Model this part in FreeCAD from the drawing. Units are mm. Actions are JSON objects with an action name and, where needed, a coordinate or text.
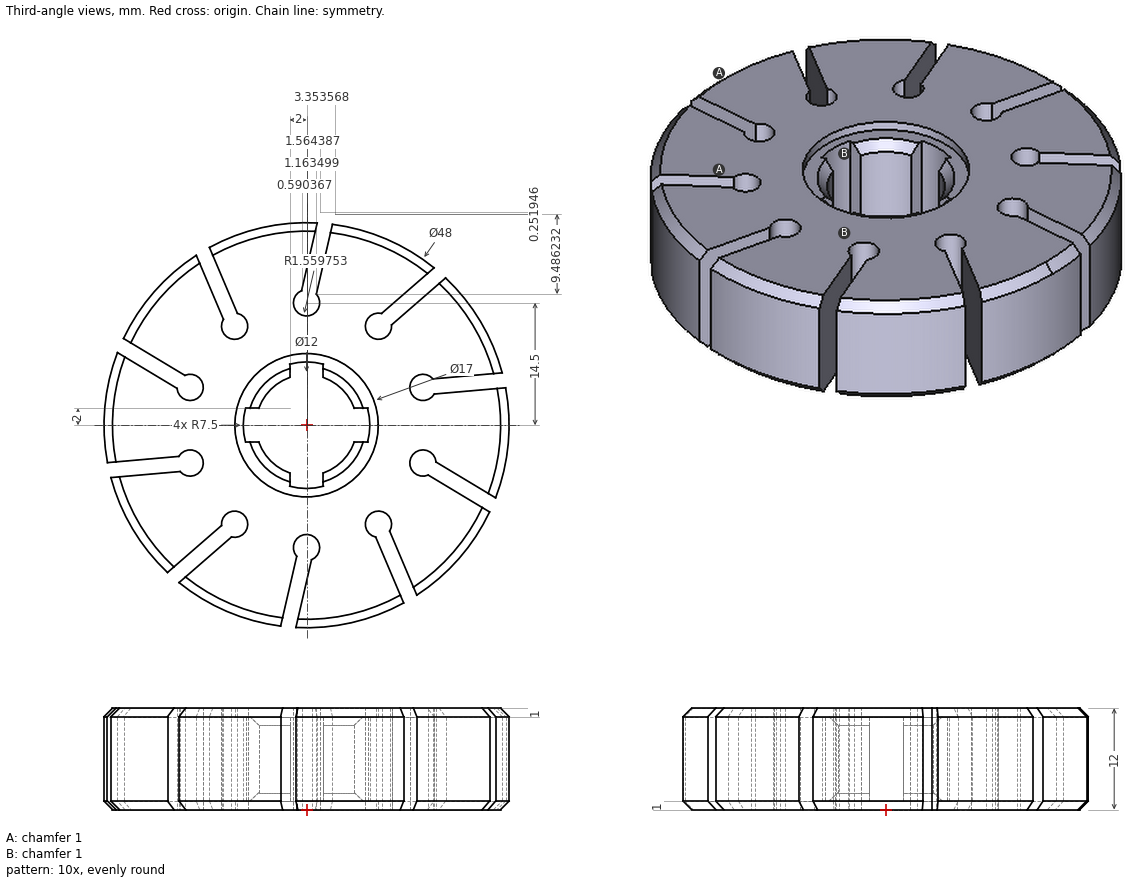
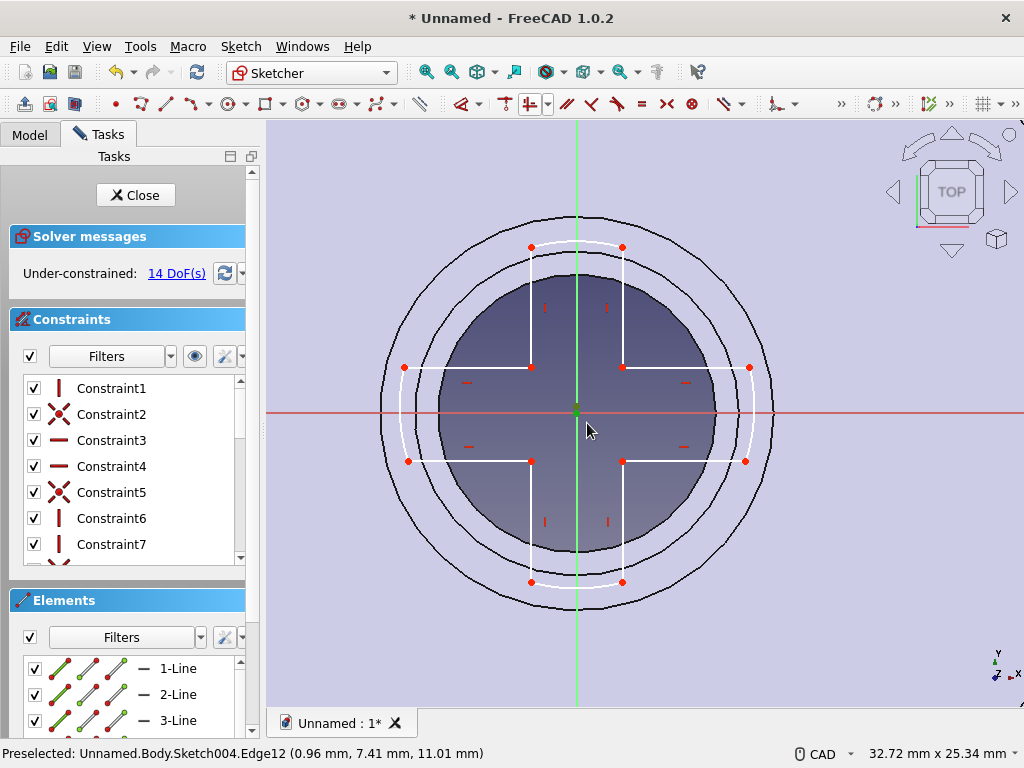
{"action": "left_click", "coordinate": [505, 104]}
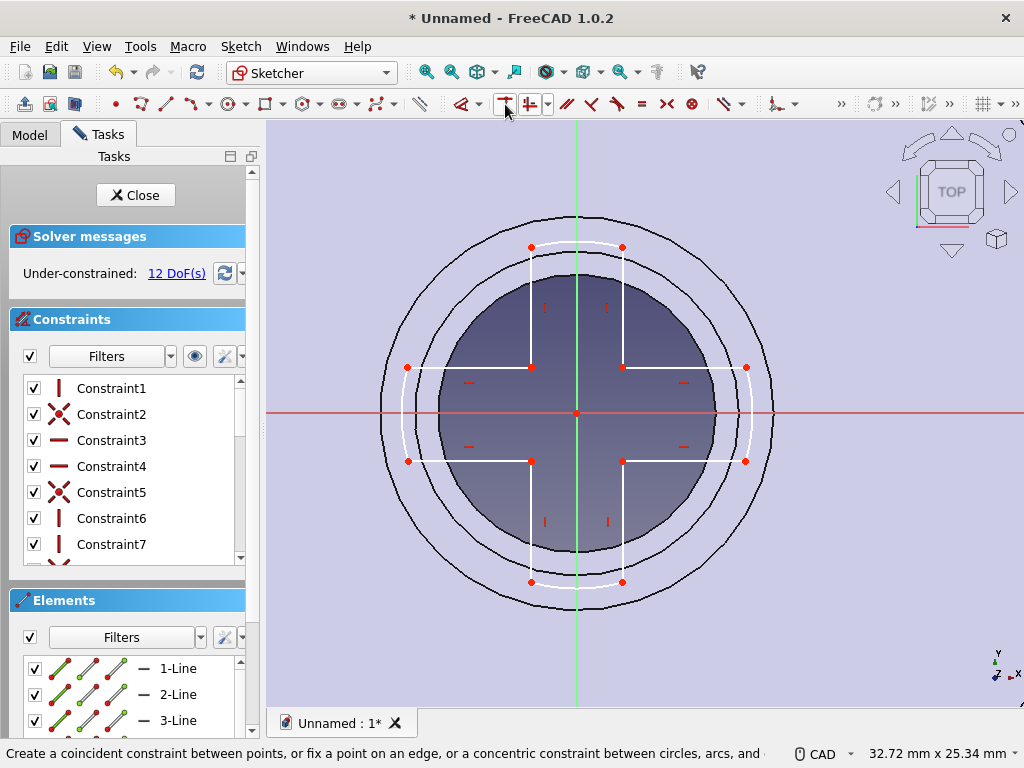
{"action": "left_click", "coordinate": [403, 396]}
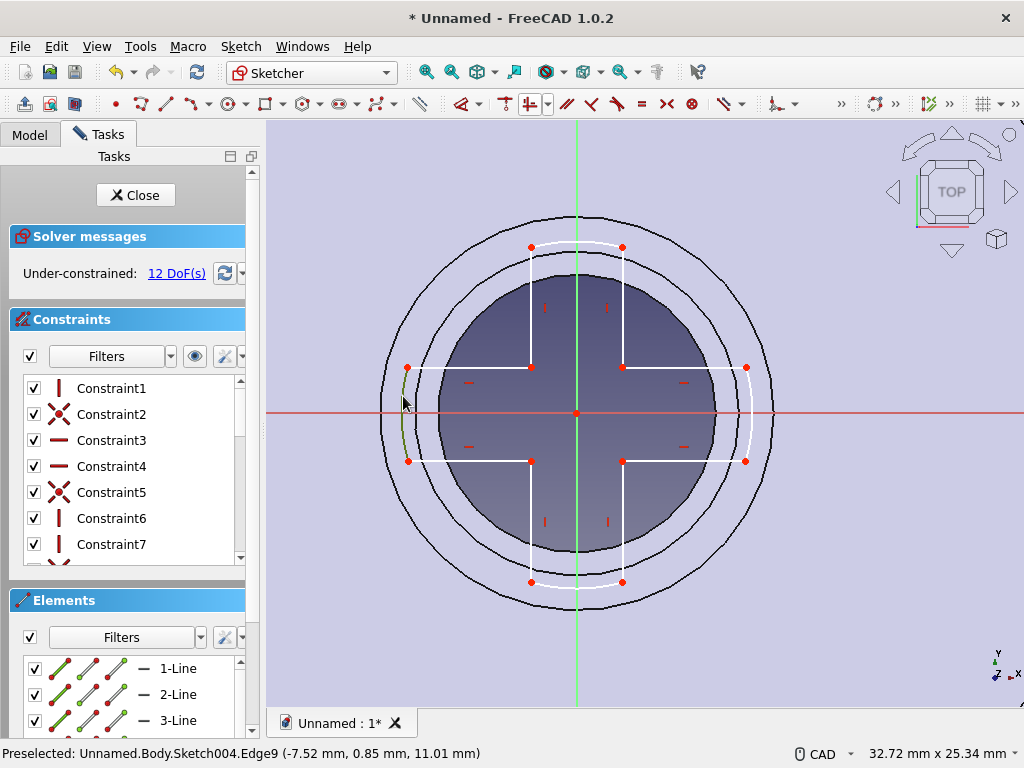
{"action": "left_click", "coordinate": [558, 588]}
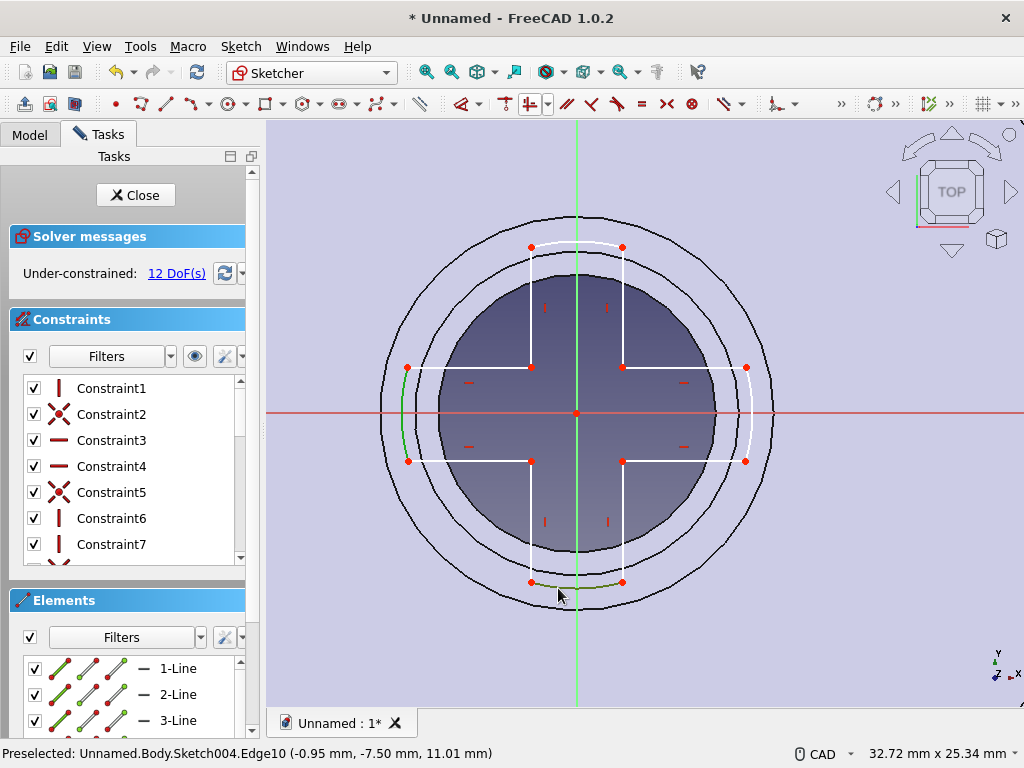
{"action": "left_click", "coordinate": [751, 433]}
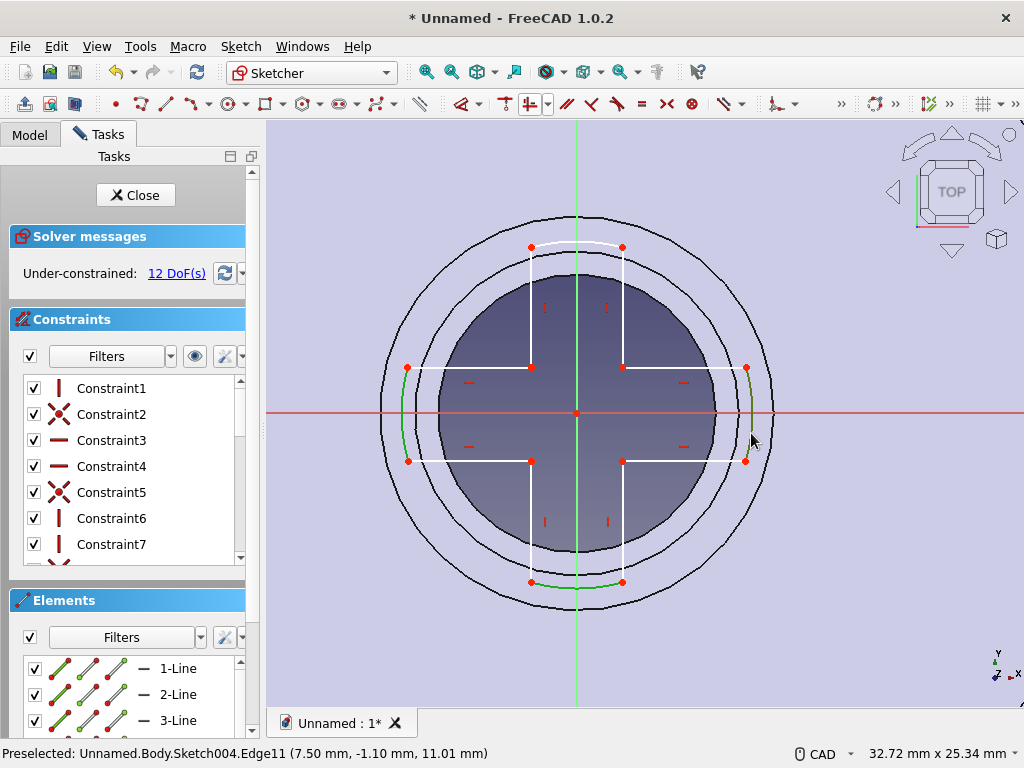
{"action": "left_click", "coordinate": [595, 243]}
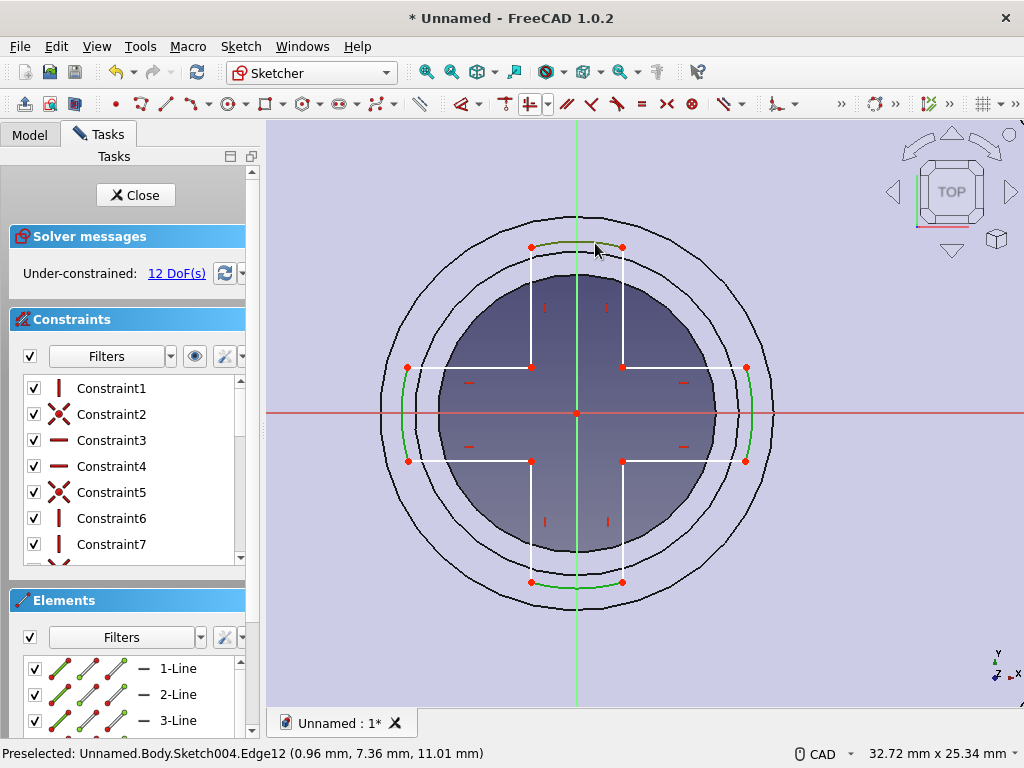
{"action": "left_click", "coordinate": [642, 104]}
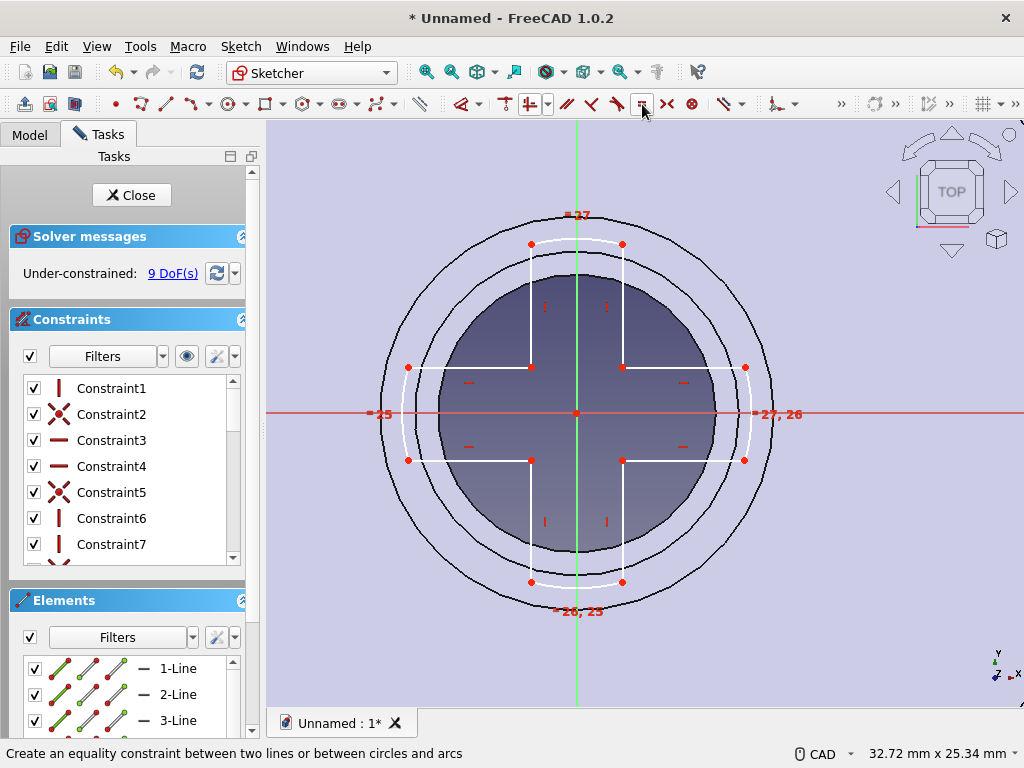
{"action": "left_click", "coordinate": [531, 368]}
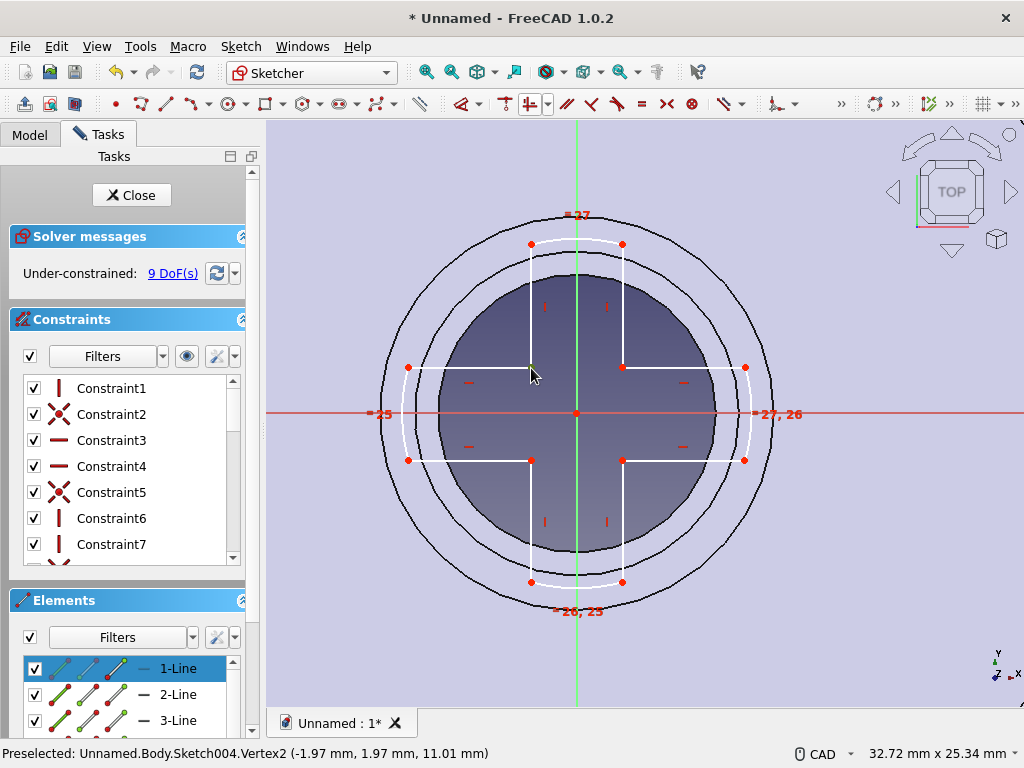
{"action": "left_click", "coordinate": [531, 461]}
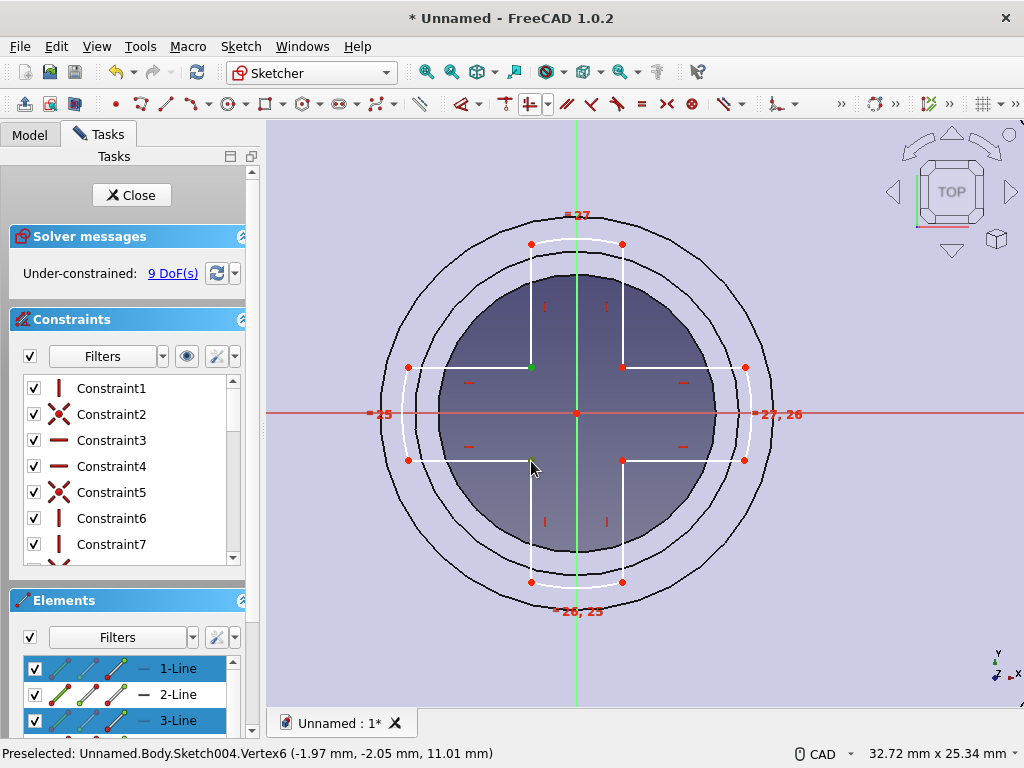
{"action": "left_click", "coordinate": [334, 413]}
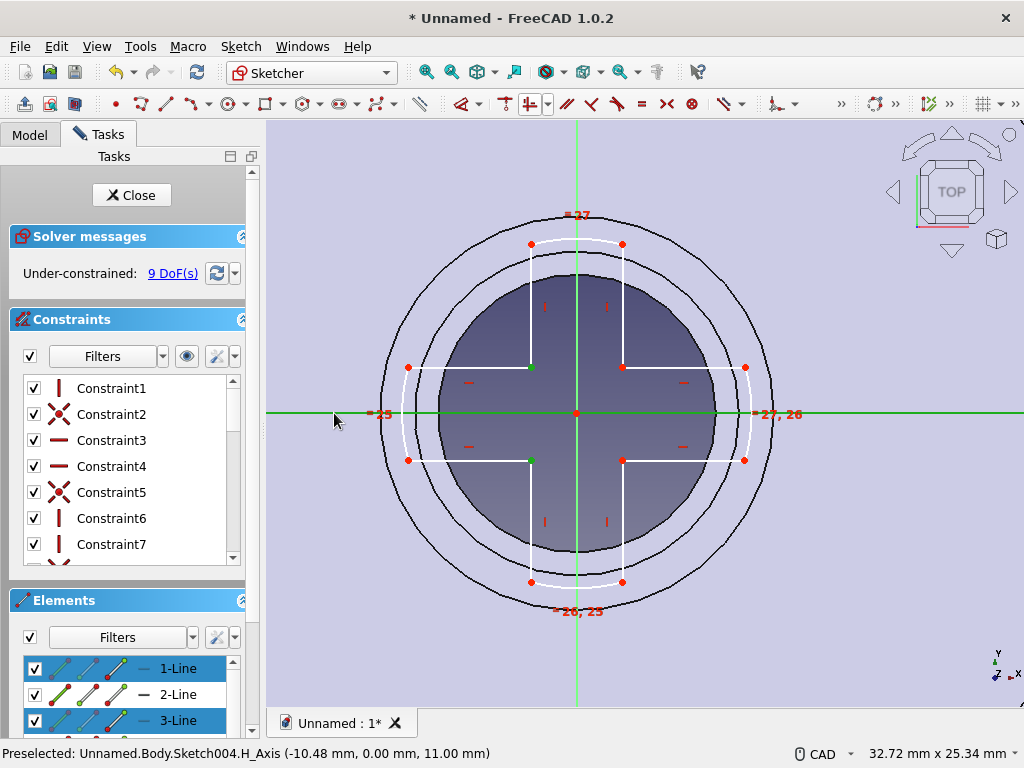
{"action": "left_click", "coordinate": [667, 104]}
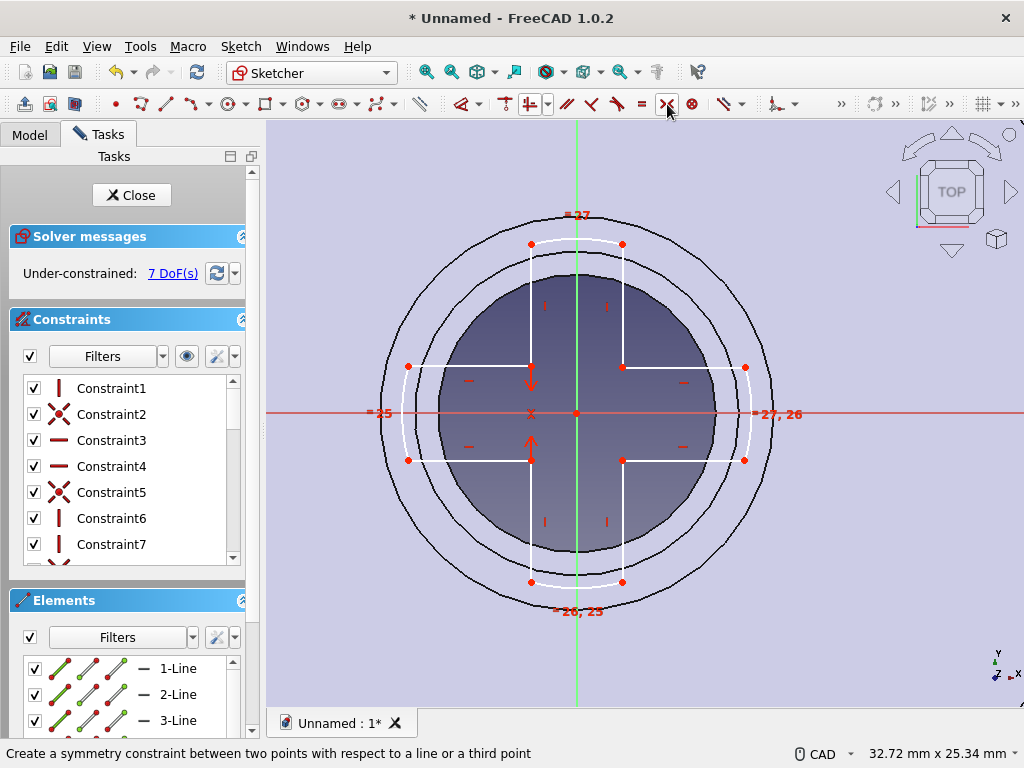
{"action": "left_click", "coordinate": [531, 461]}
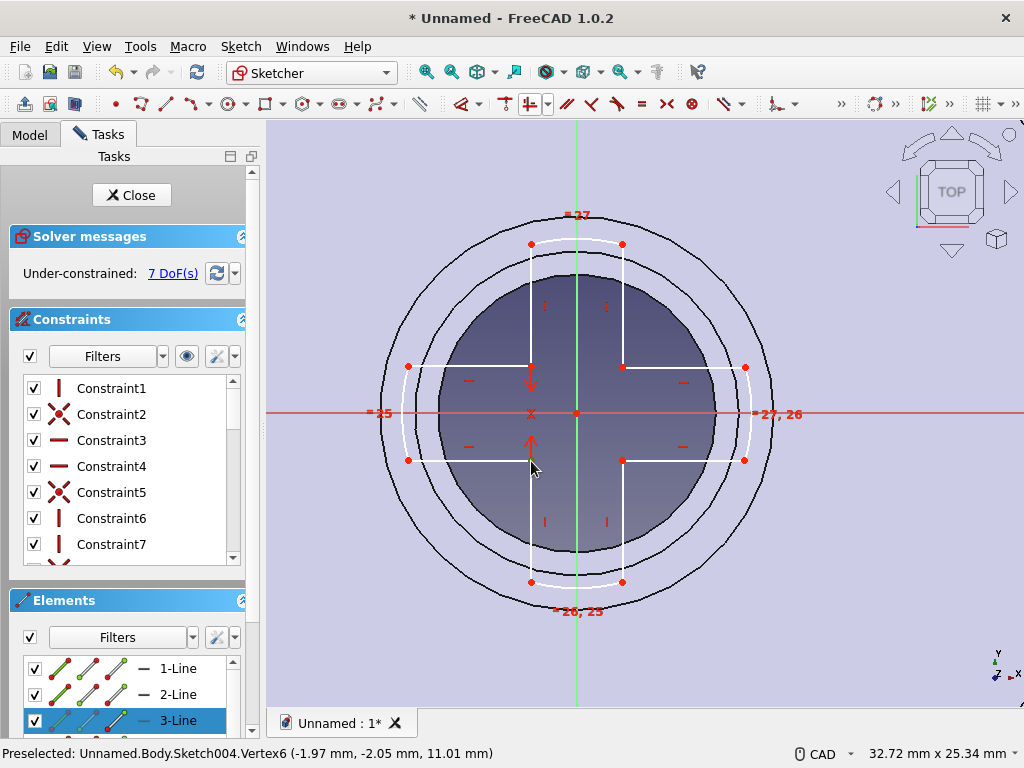
{"action": "left_click", "coordinate": [623, 461]}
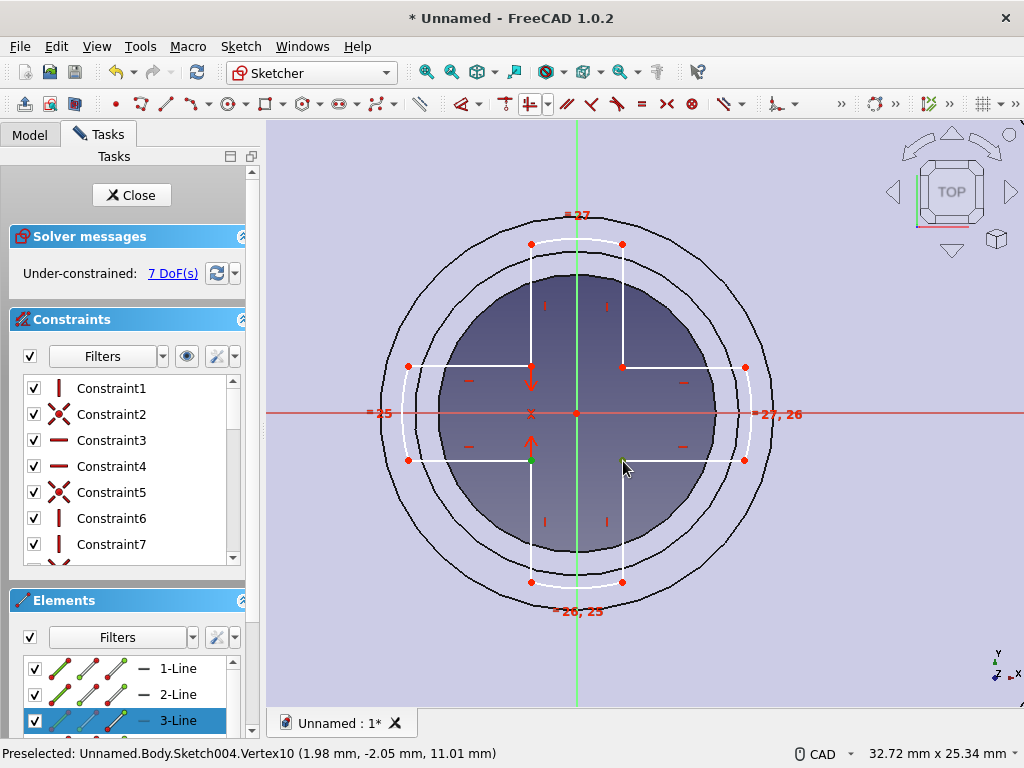
{"action": "left_click", "coordinate": [577, 641]}